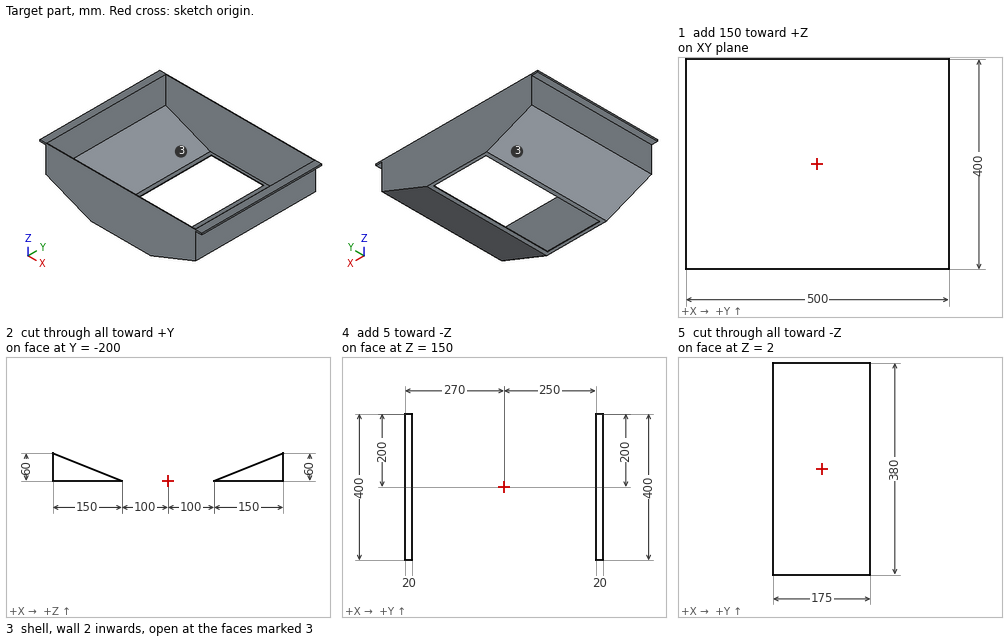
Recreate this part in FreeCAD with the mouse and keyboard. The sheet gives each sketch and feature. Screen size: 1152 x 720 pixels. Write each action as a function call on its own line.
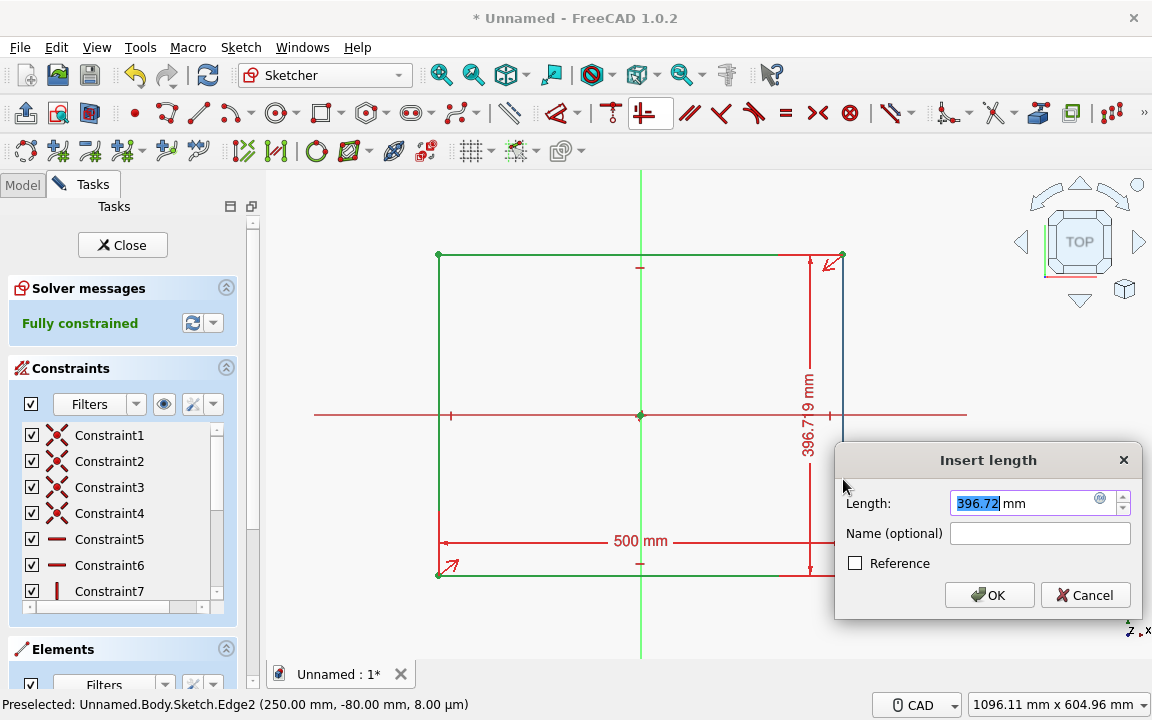
text(400)
key(Return)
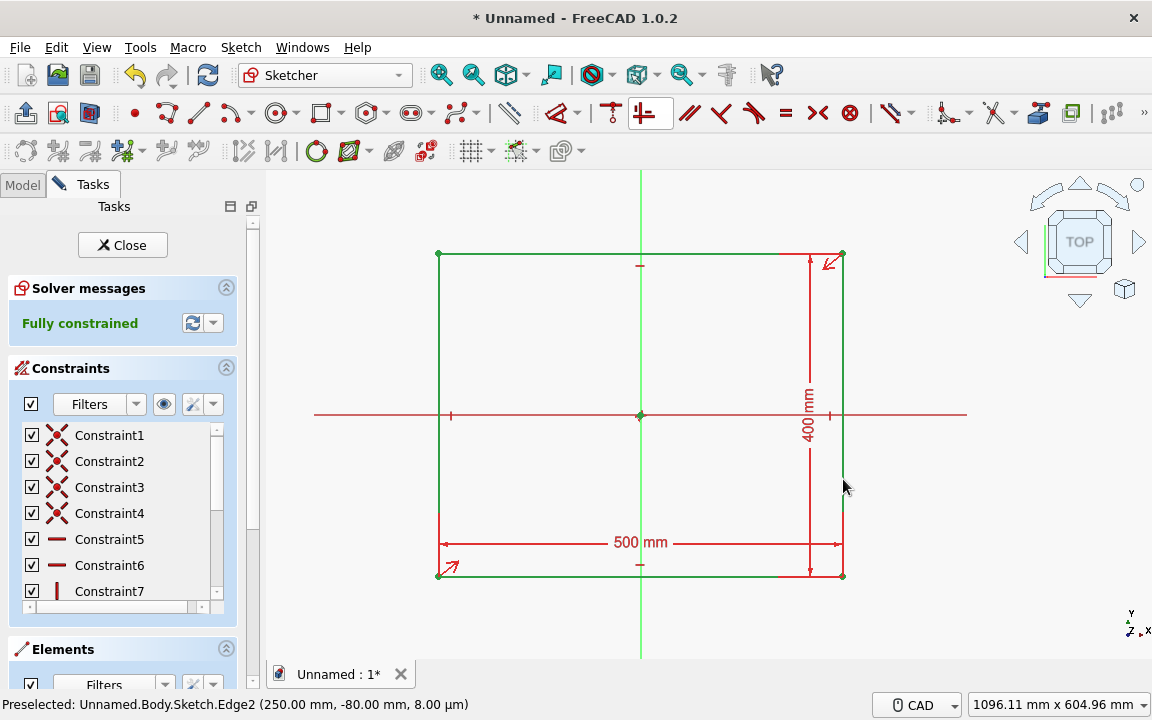
click(123, 245)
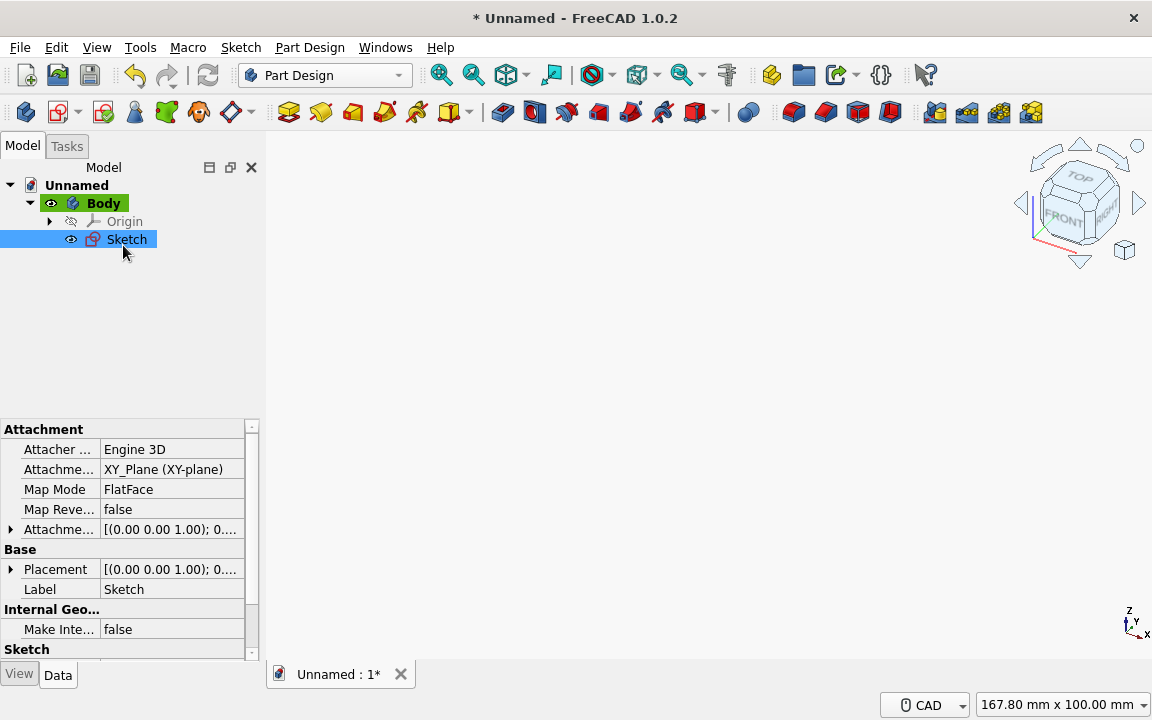
click(290, 112)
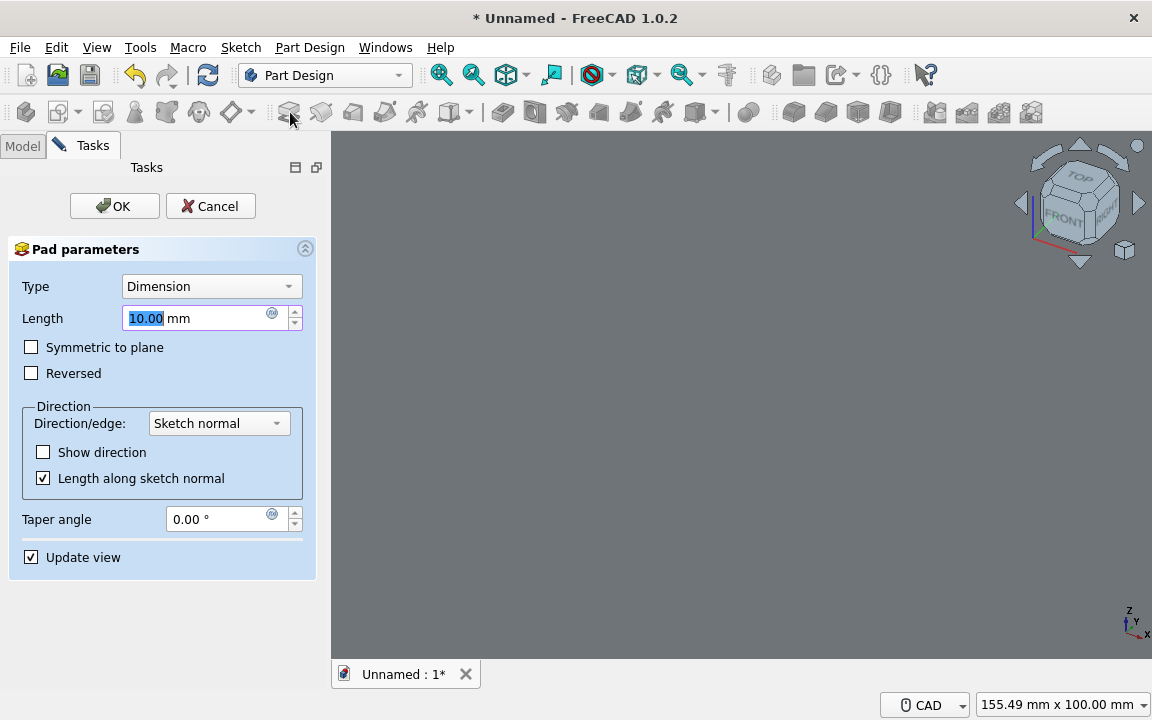
text(150)
key(Tab)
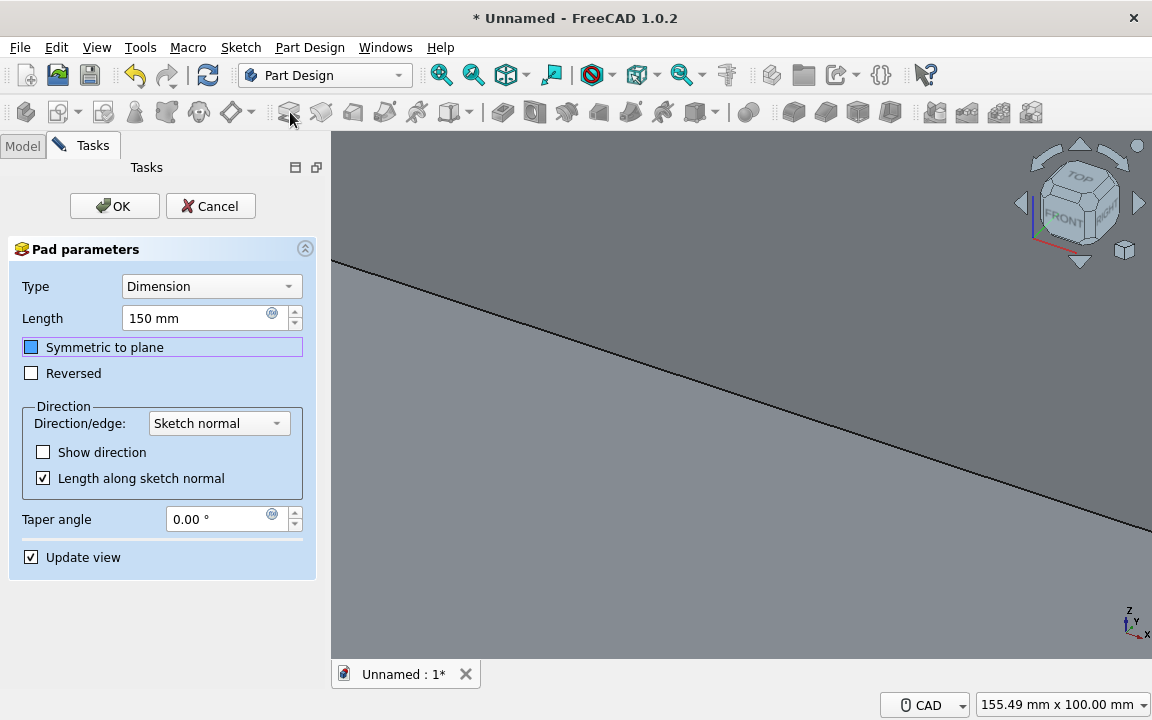
click(115, 206)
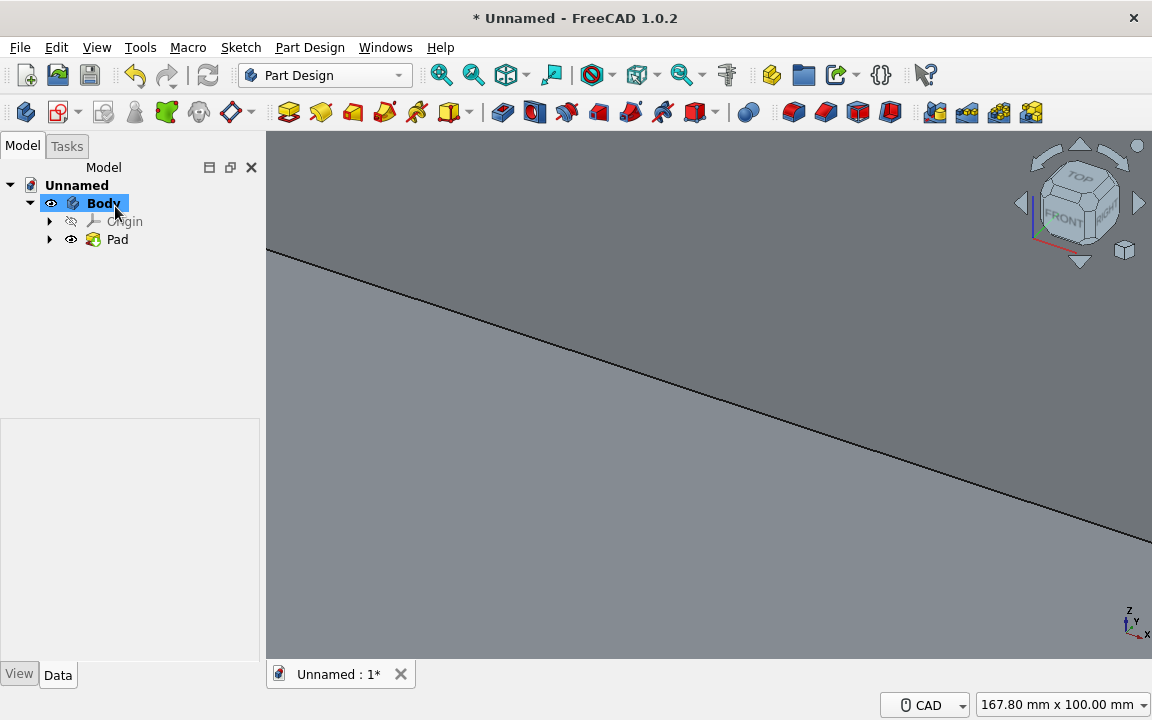
click(442, 76)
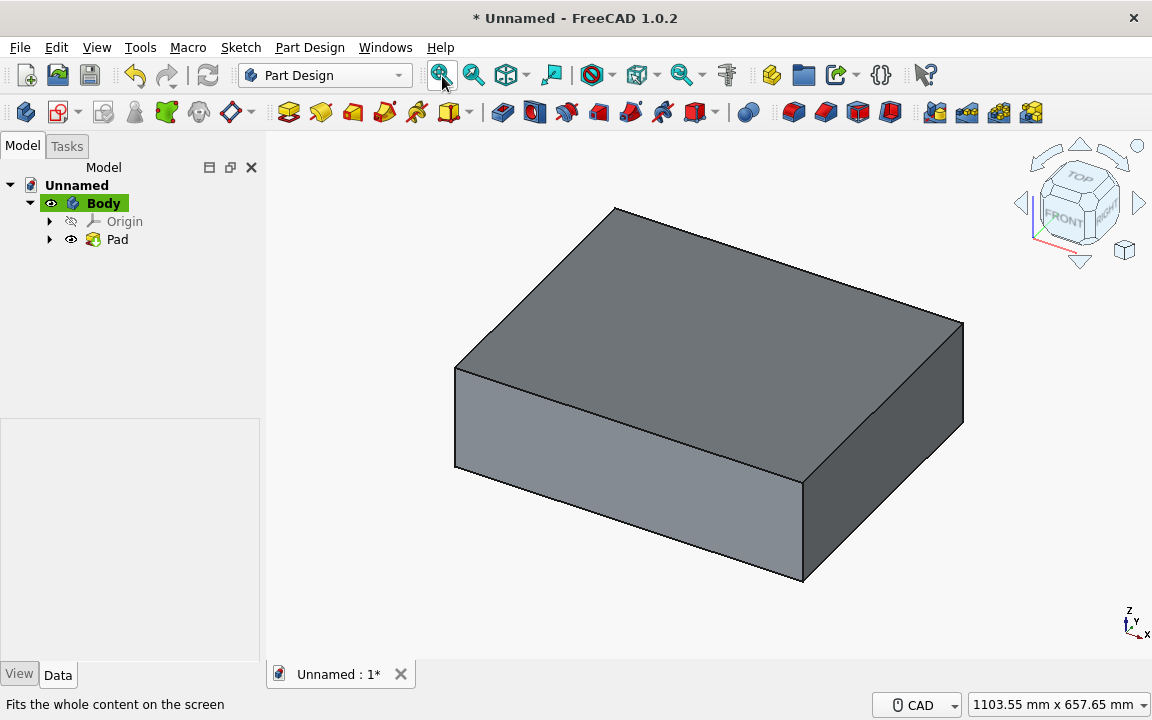
click(728, 507)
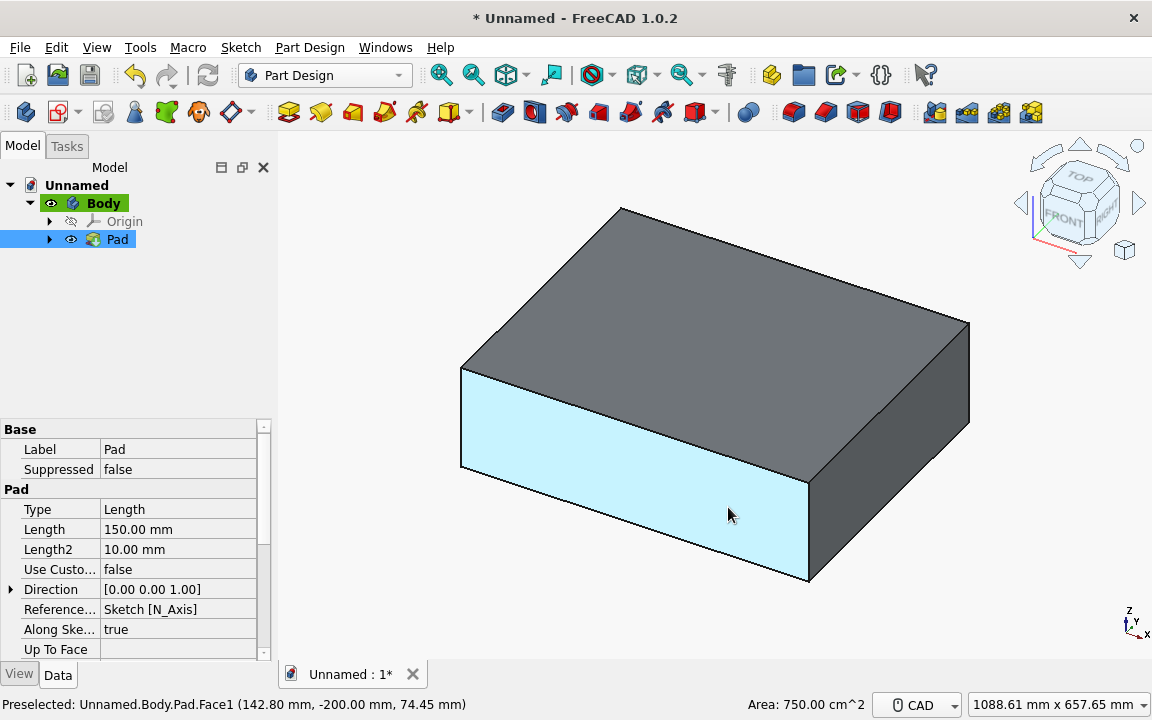
click(58, 112)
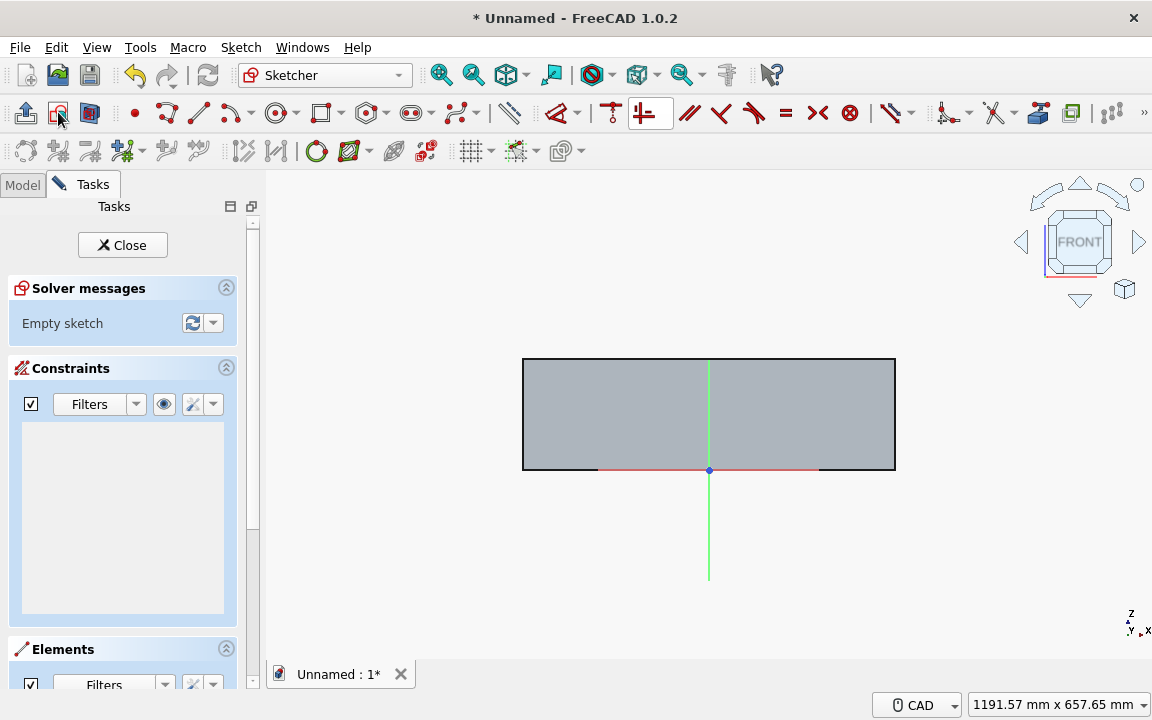
key(g)
key(m)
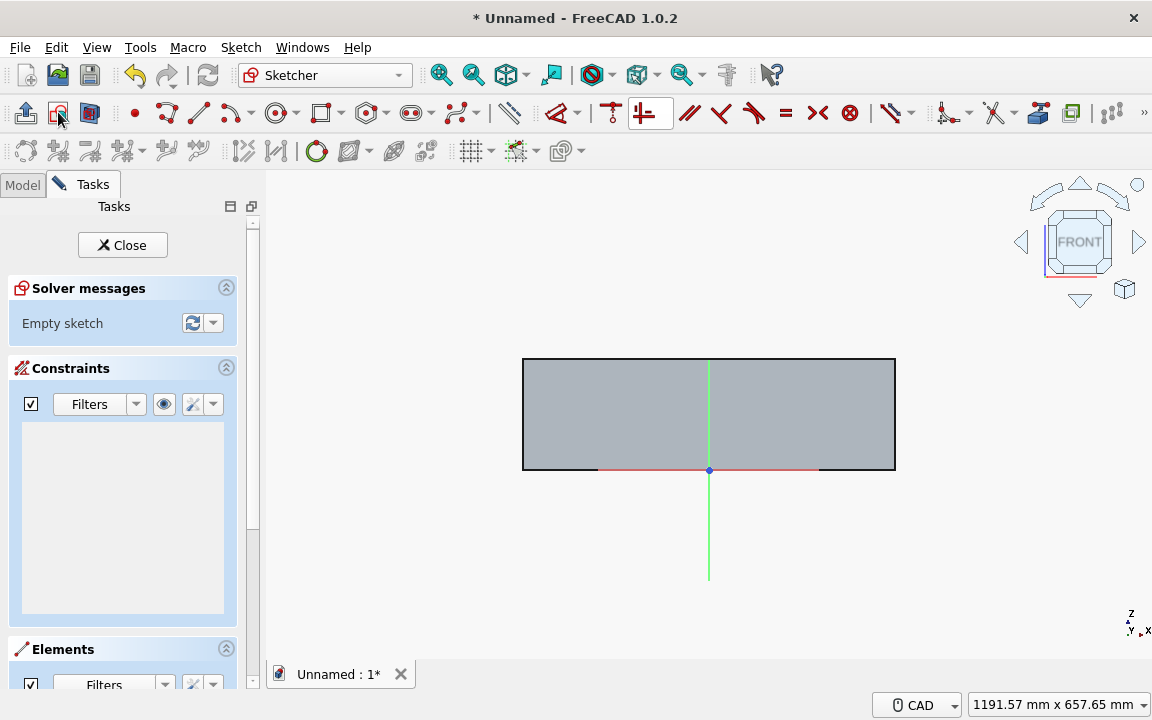
click(635, 470)
click(523, 426)
click(523, 461)
click(635, 470)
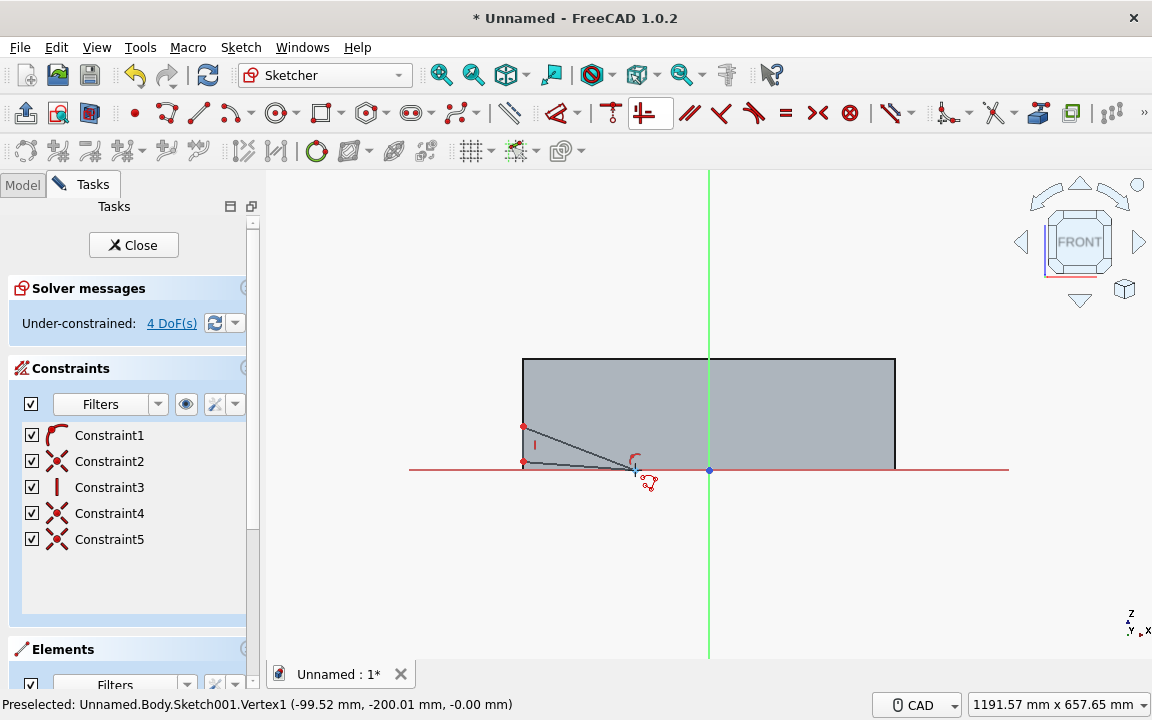
click(783, 470)
click(895, 461)
click(895, 426)
click(783, 470)
key(Escape)
key(Escape)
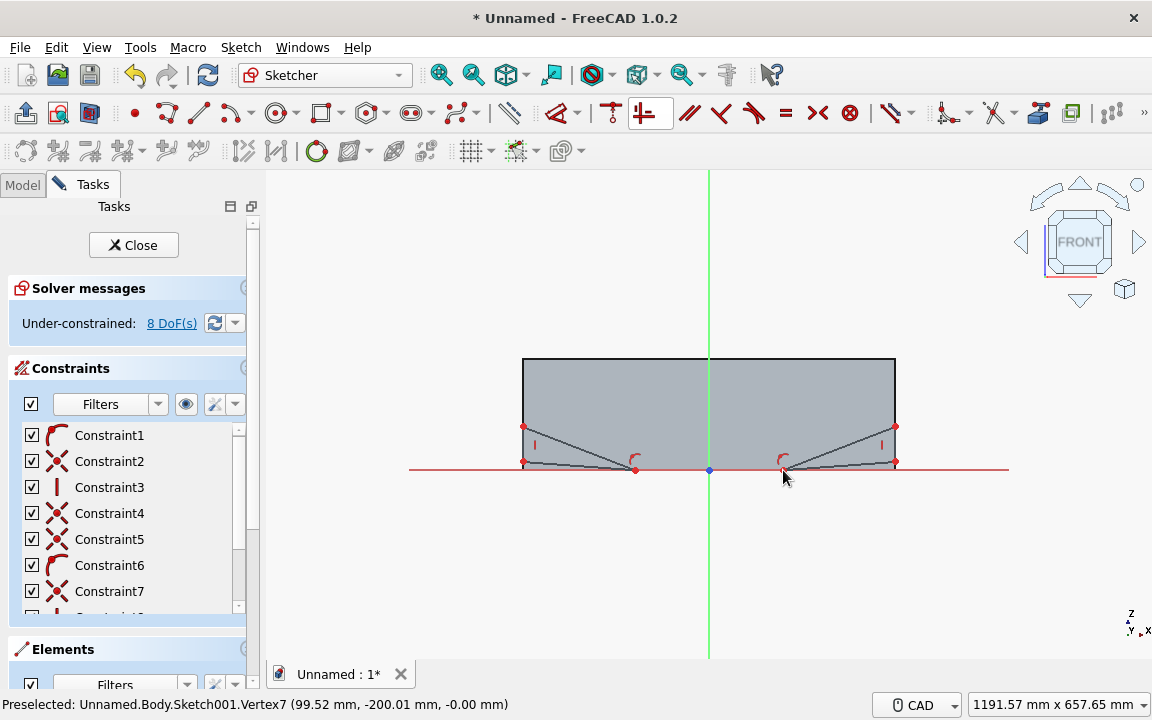
scroll(601, 468, up, 2)